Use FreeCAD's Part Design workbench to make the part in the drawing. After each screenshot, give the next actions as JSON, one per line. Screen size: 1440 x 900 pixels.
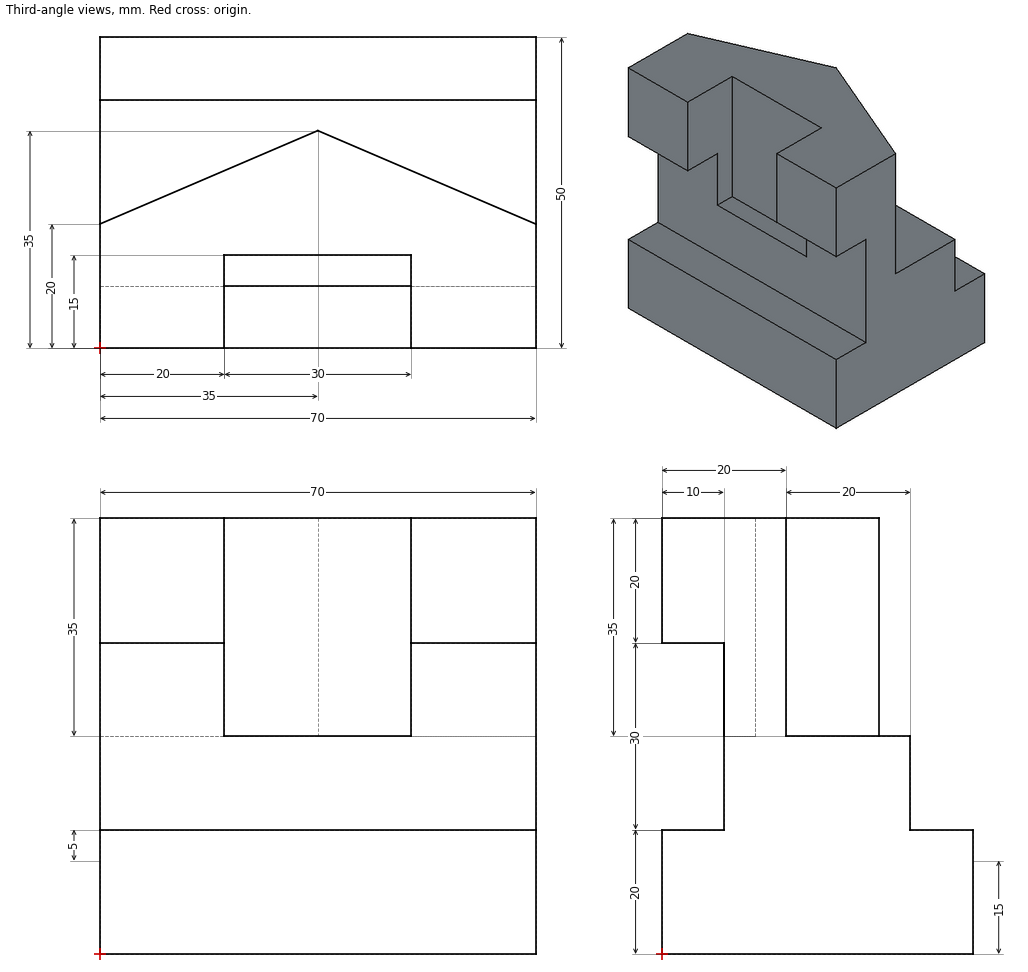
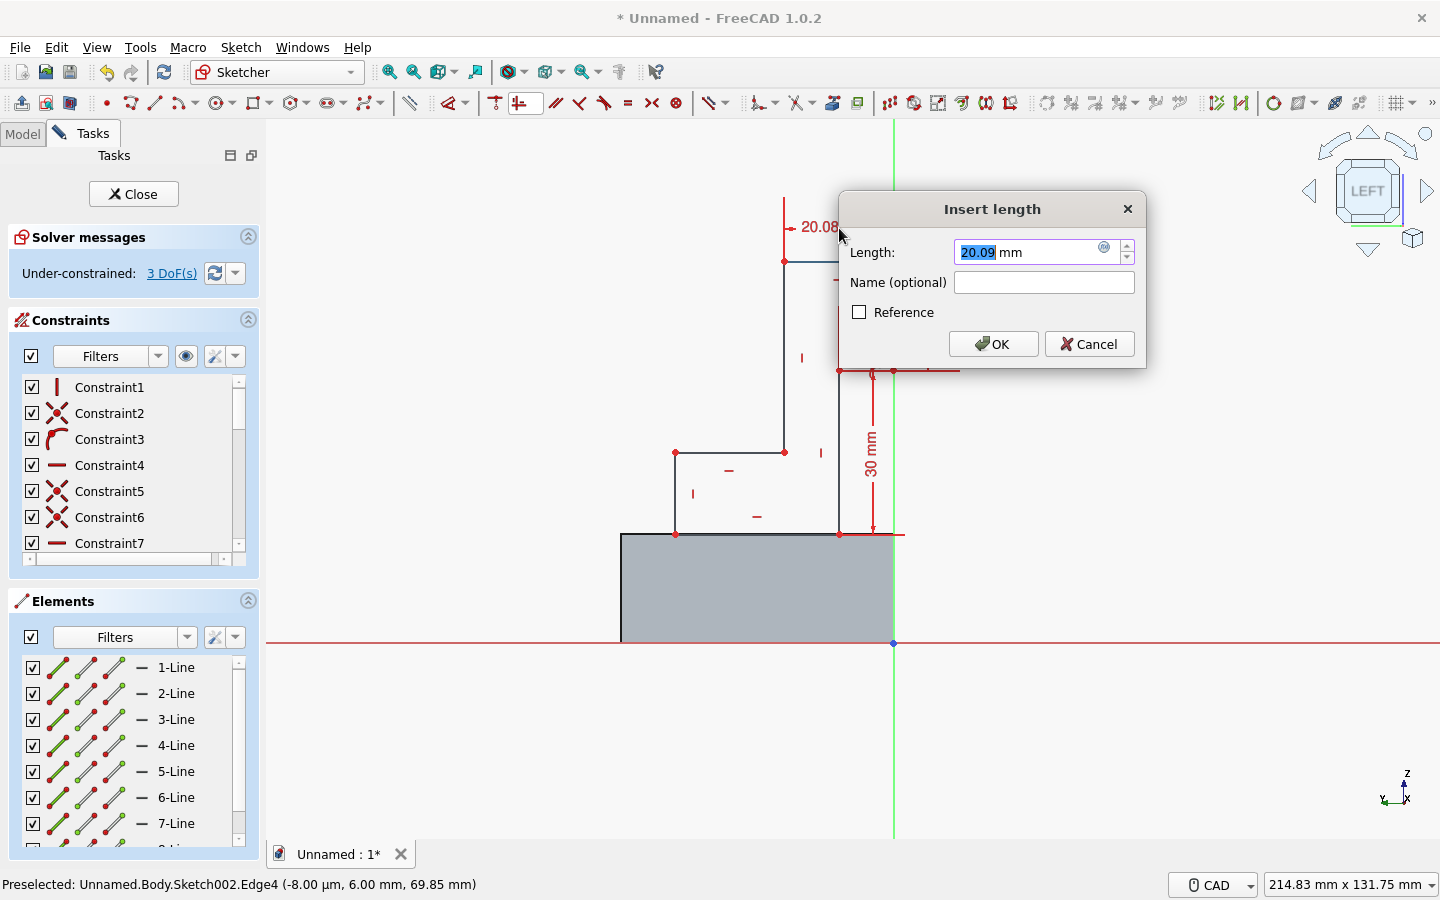
{"action": "type", "text": "20"}
{"action": "key", "text": "Return"}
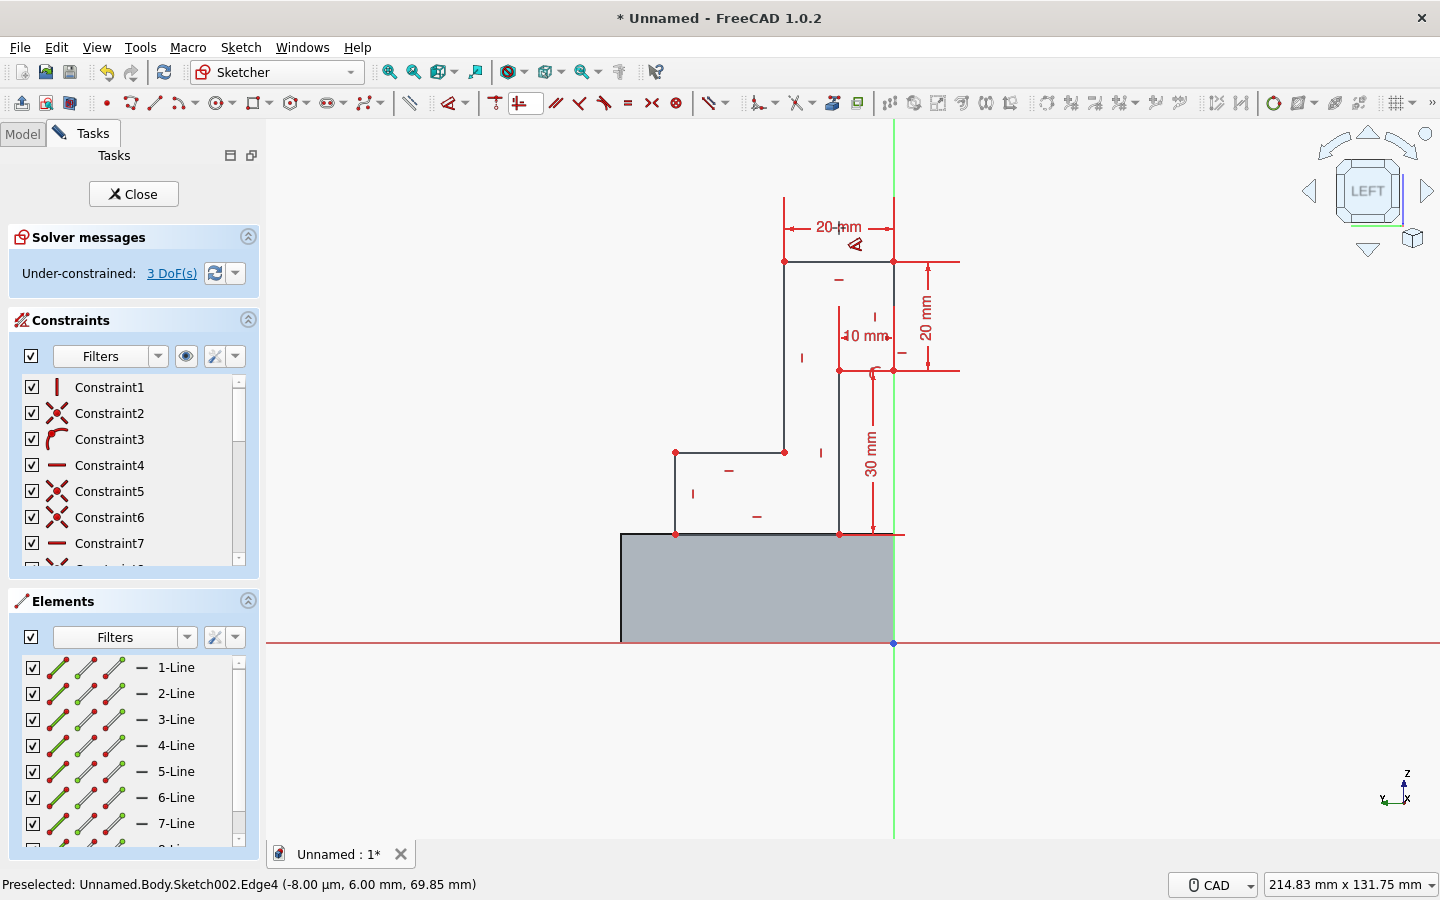
{"action": "left_click", "coordinate": [784, 319]}
{"action": "left_click", "coordinate": [818, 357]}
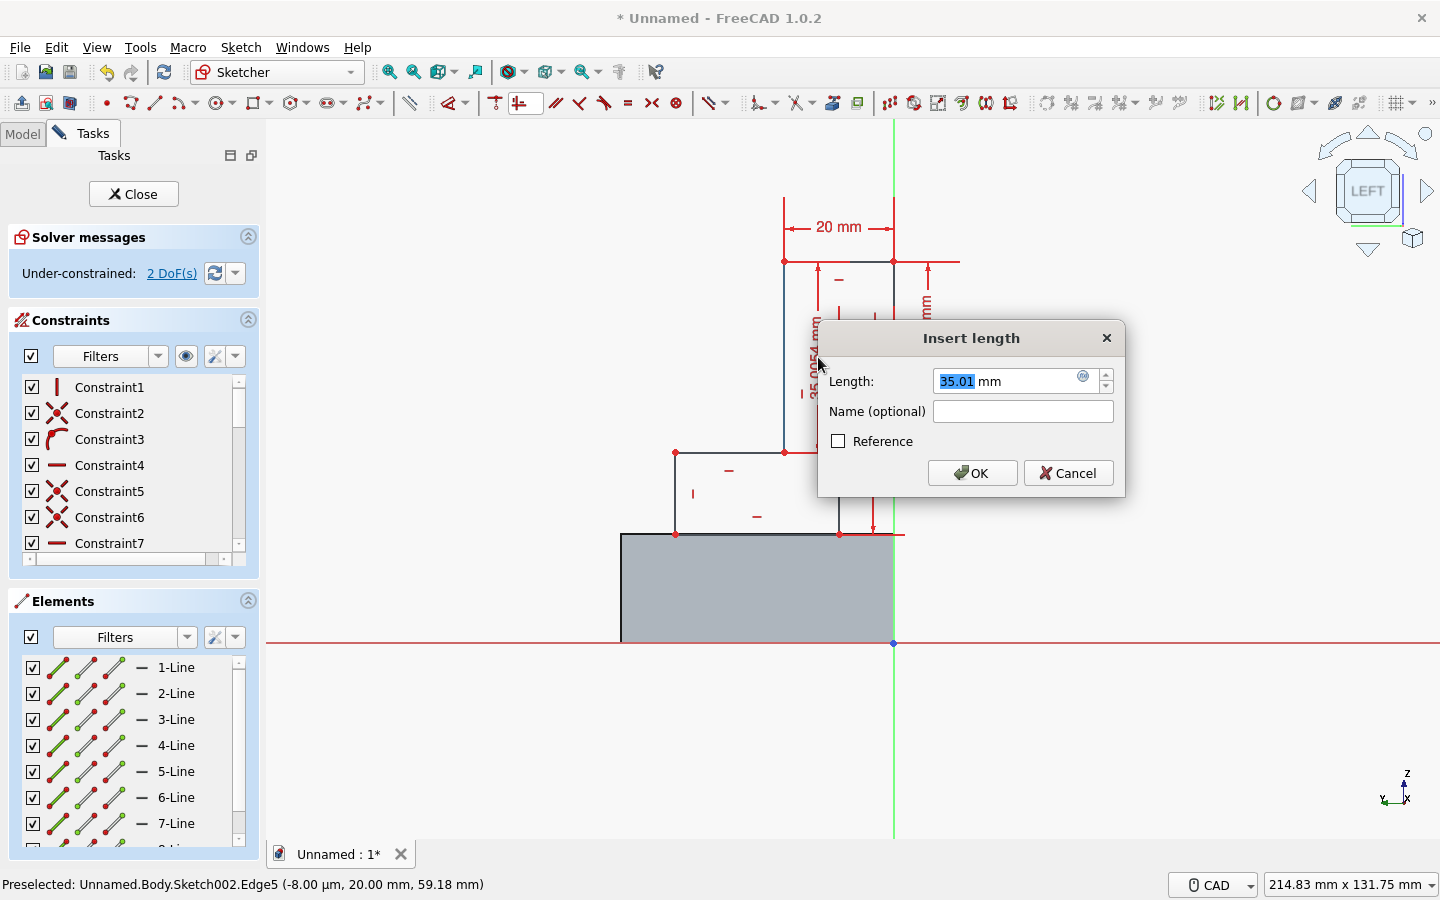
{"action": "type", "text": "35"}
{"action": "key", "text": "Return"}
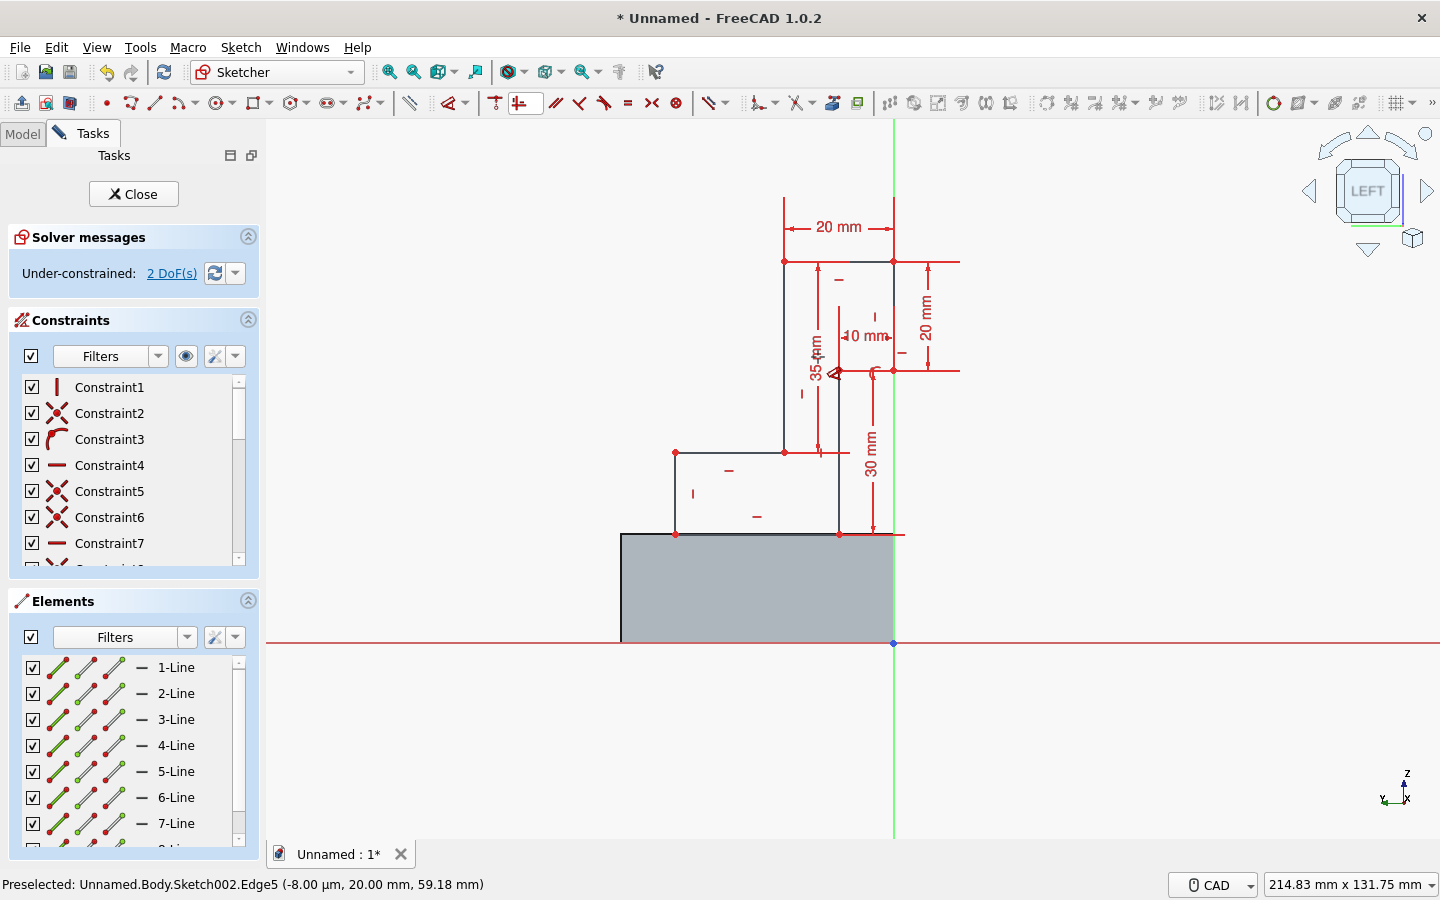
{"action": "left_click", "coordinate": [752, 453]}
{"action": "left_click", "coordinate": [730, 487]}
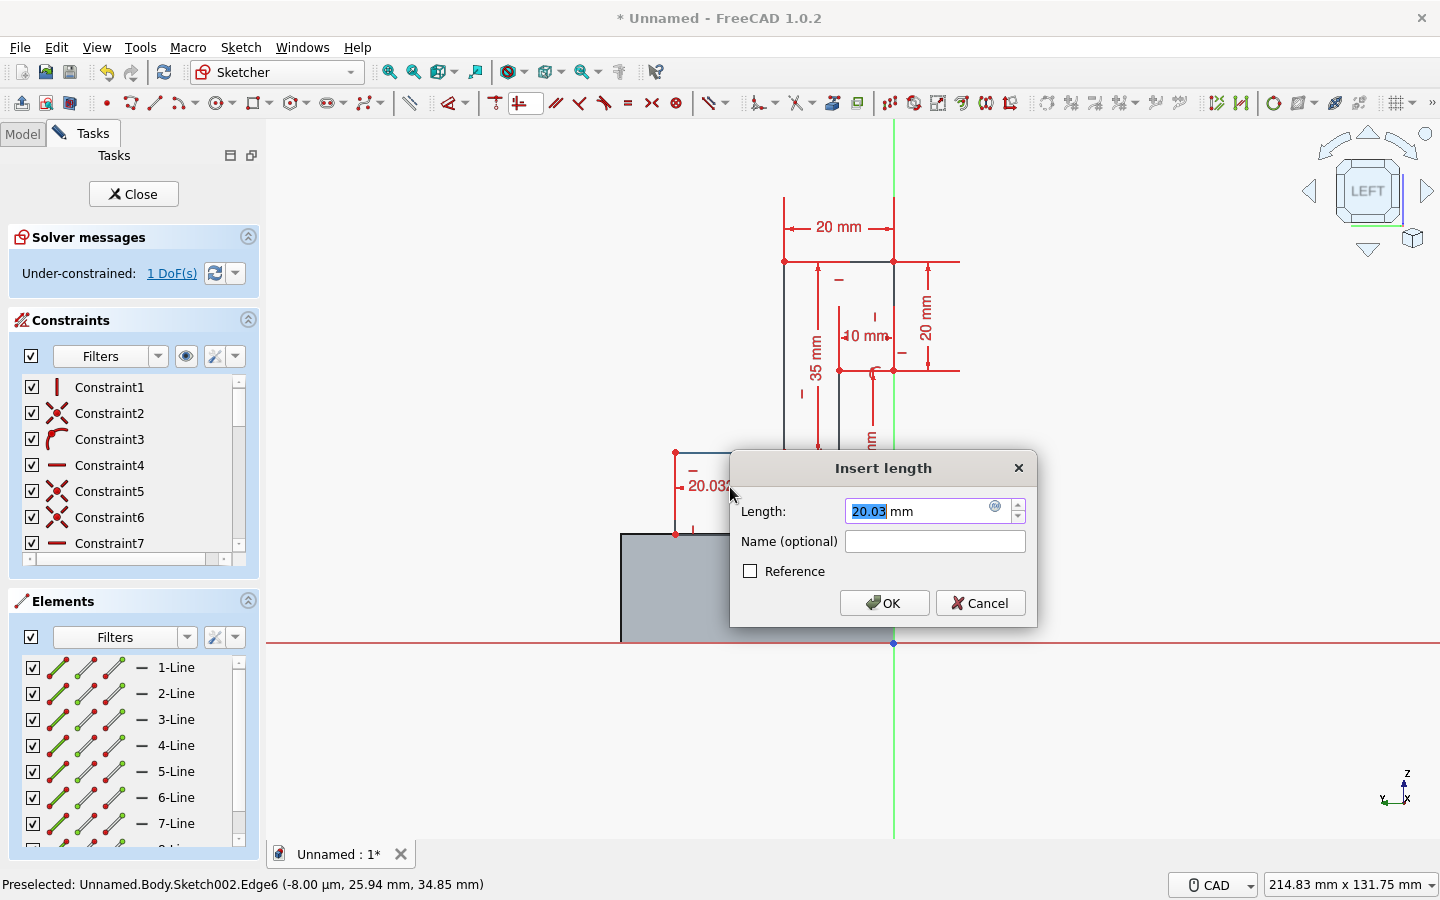
{"action": "type", "text": "20"}
{"action": "key", "text": "Return"}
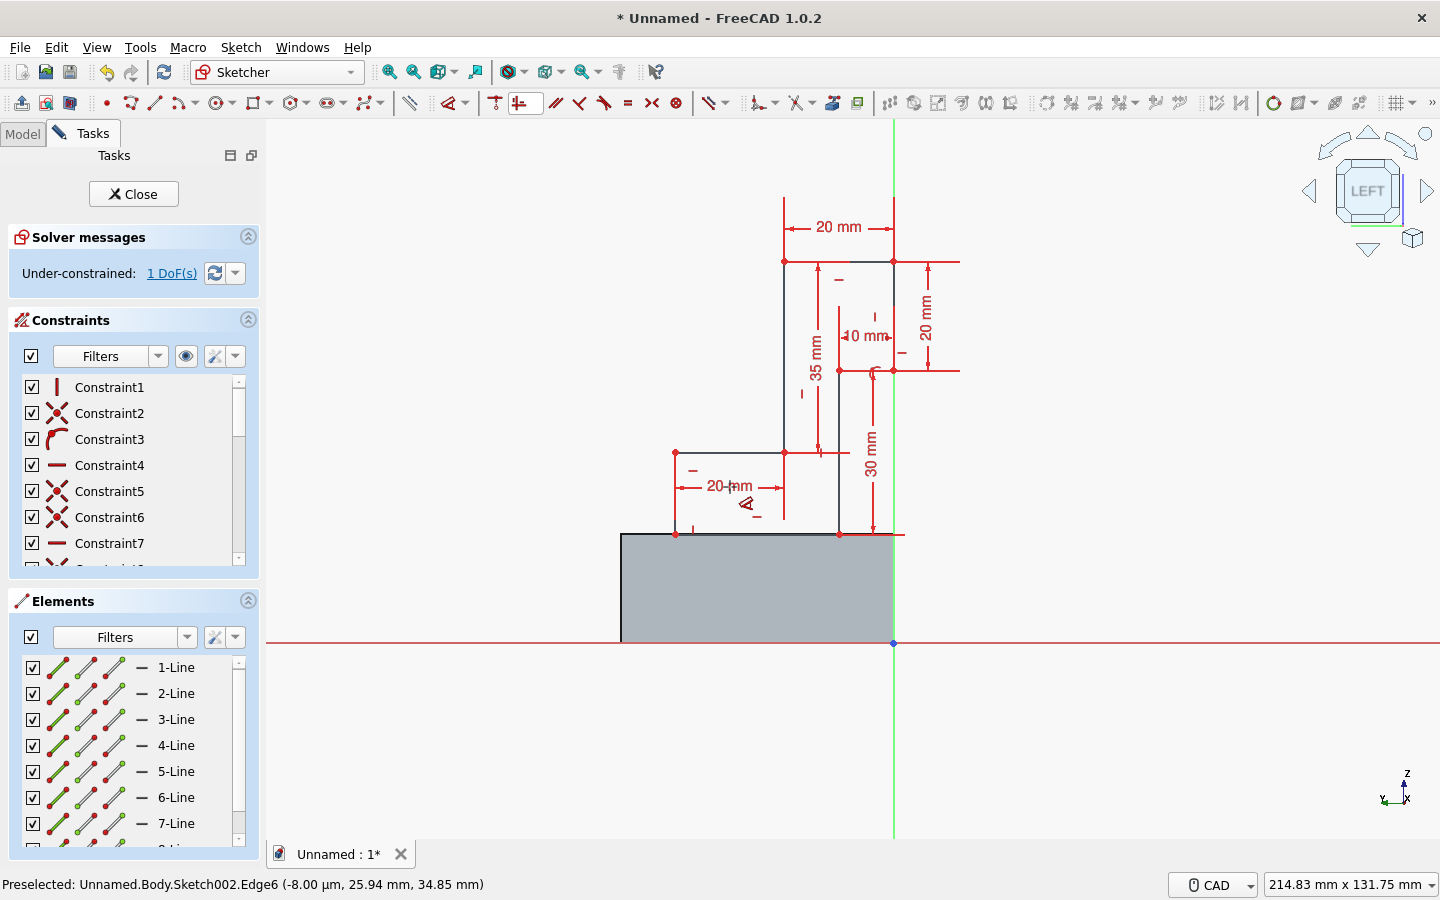
{"action": "left_click", "coordinate": [839, 535]}
{"action": "left_click", "coordinate": [928, 589]}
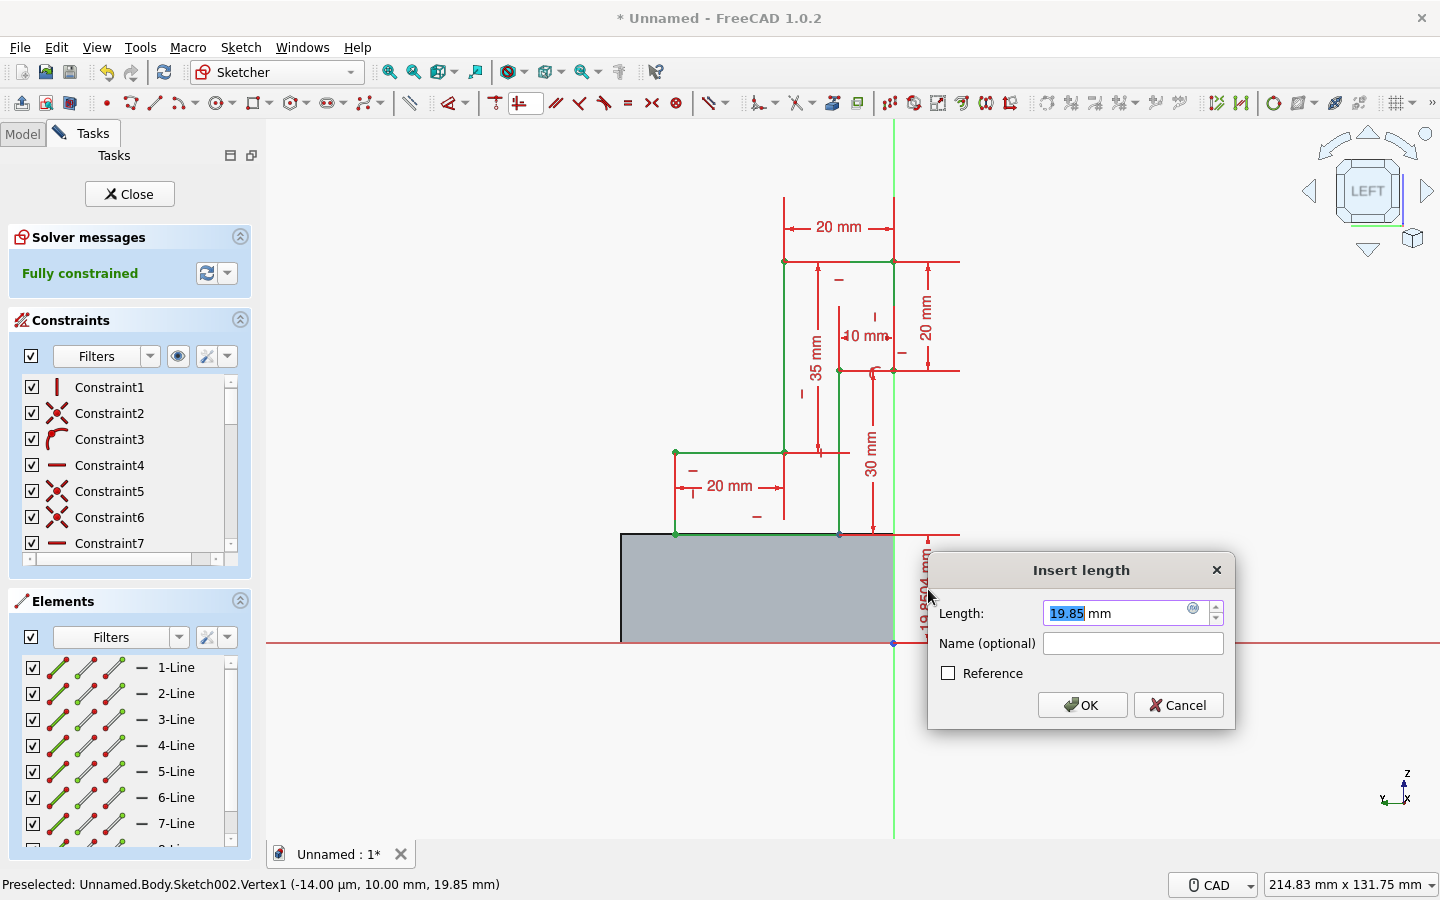
{"action": "type", "text": "20"}
{"action": "key", "text": "Return"}
{"action": "key", "text": "Escape"}